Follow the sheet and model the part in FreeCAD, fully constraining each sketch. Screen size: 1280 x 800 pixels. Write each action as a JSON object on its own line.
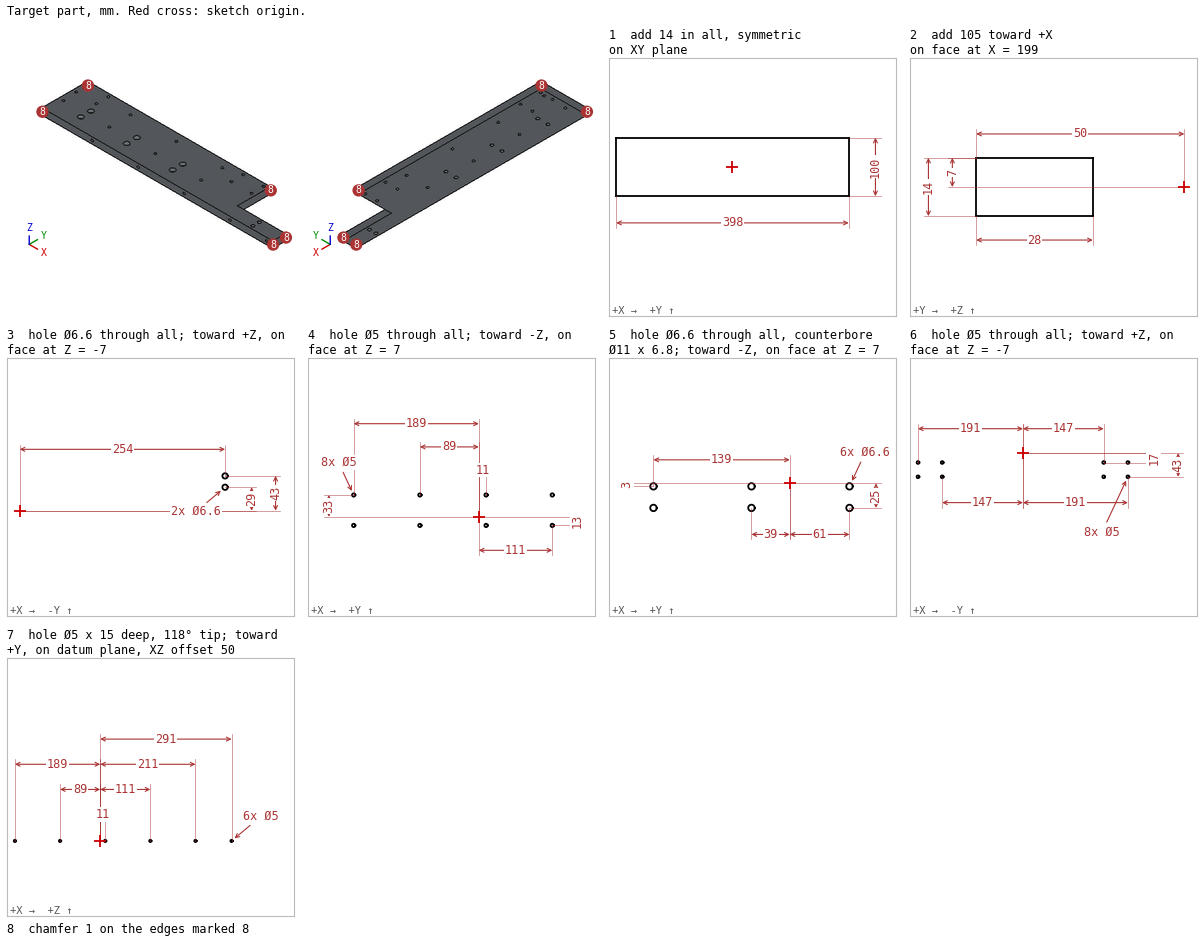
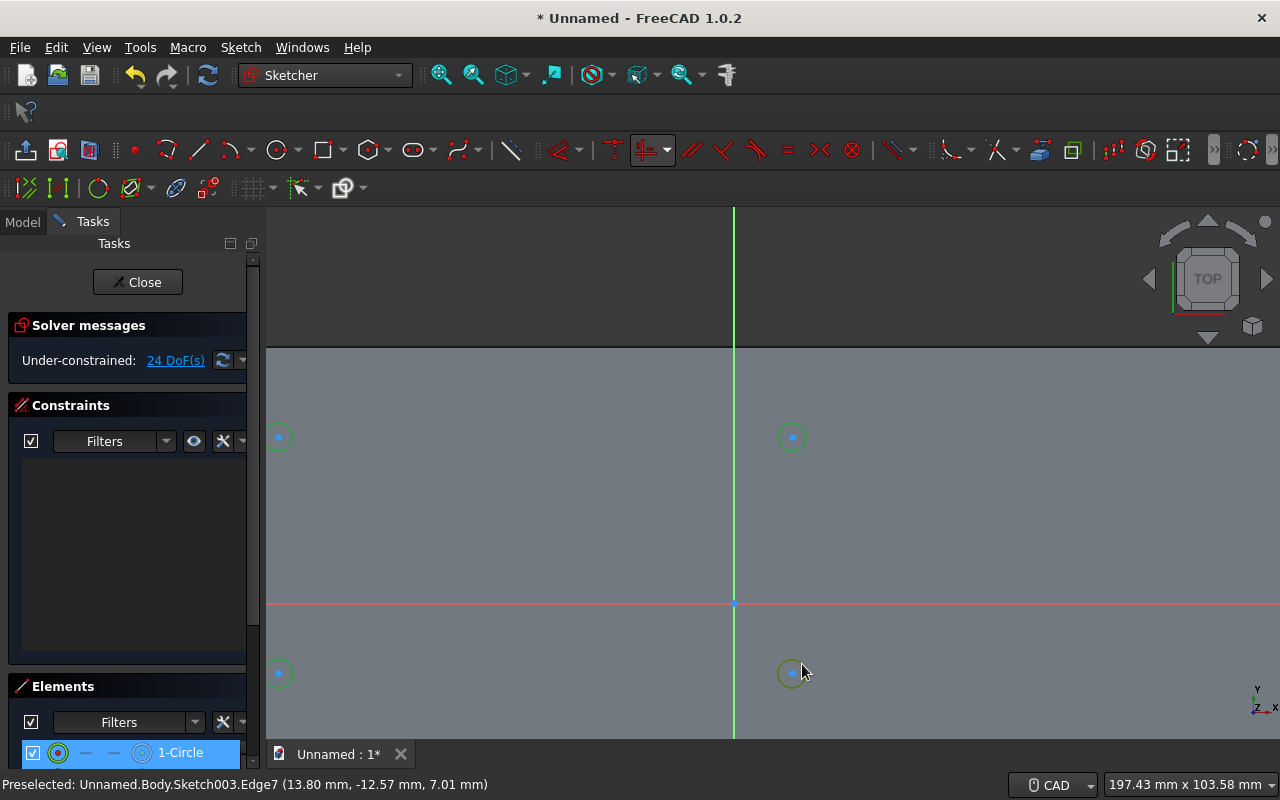
{"action": "scroll", "coordinate": [804, 427], "scroll_direction": "down", "scroll_amount": 5}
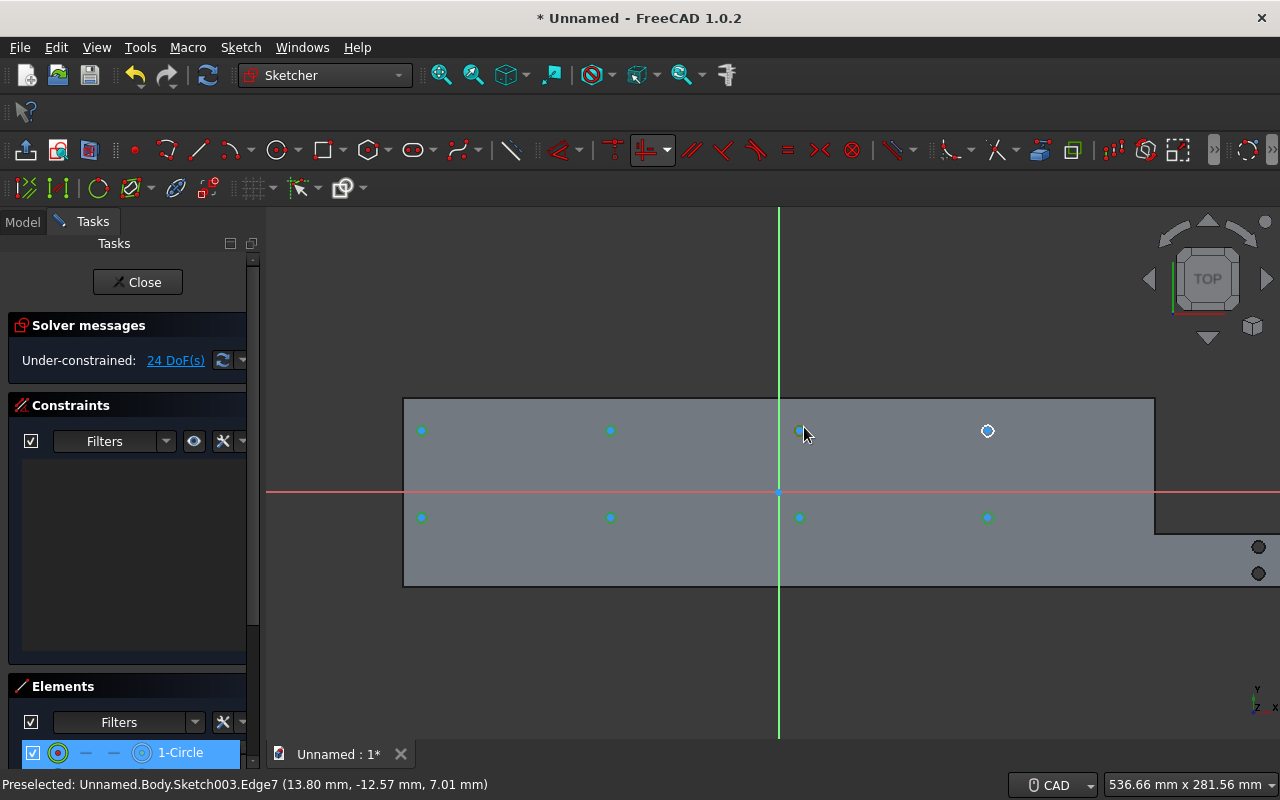
{"action": "scroll", "coordinate": [992, 427], "scroll_direction": "up", "scroll_amount": 5}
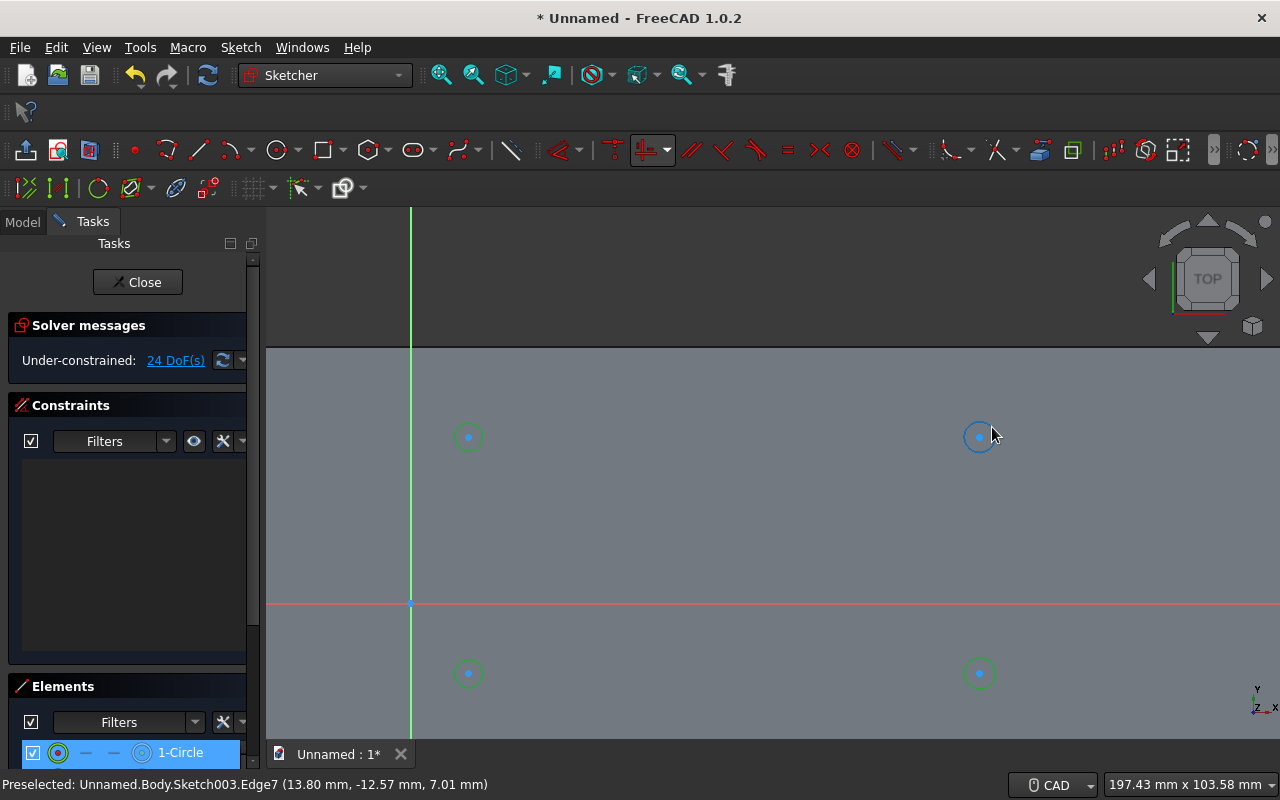
{"action": "left_click", "coordinate": [991, 426]}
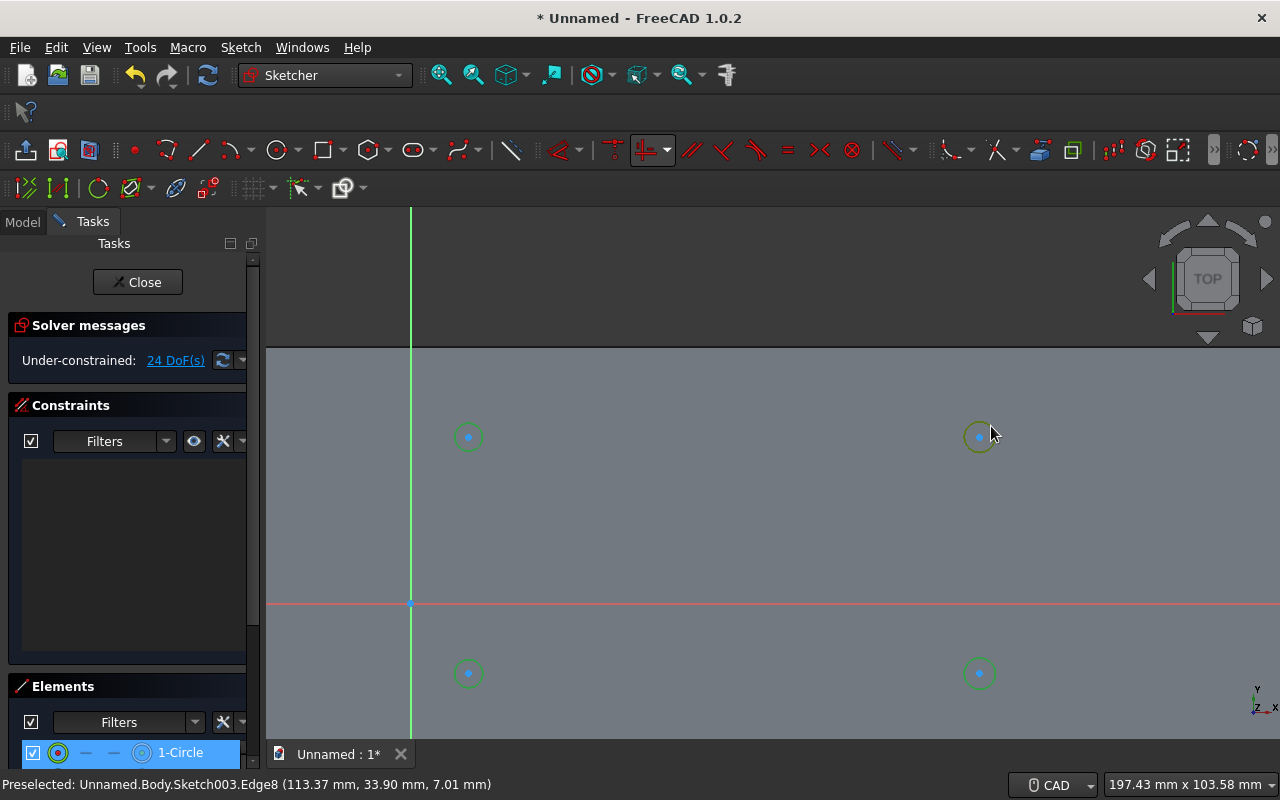
{"action": "key", "text": "e"}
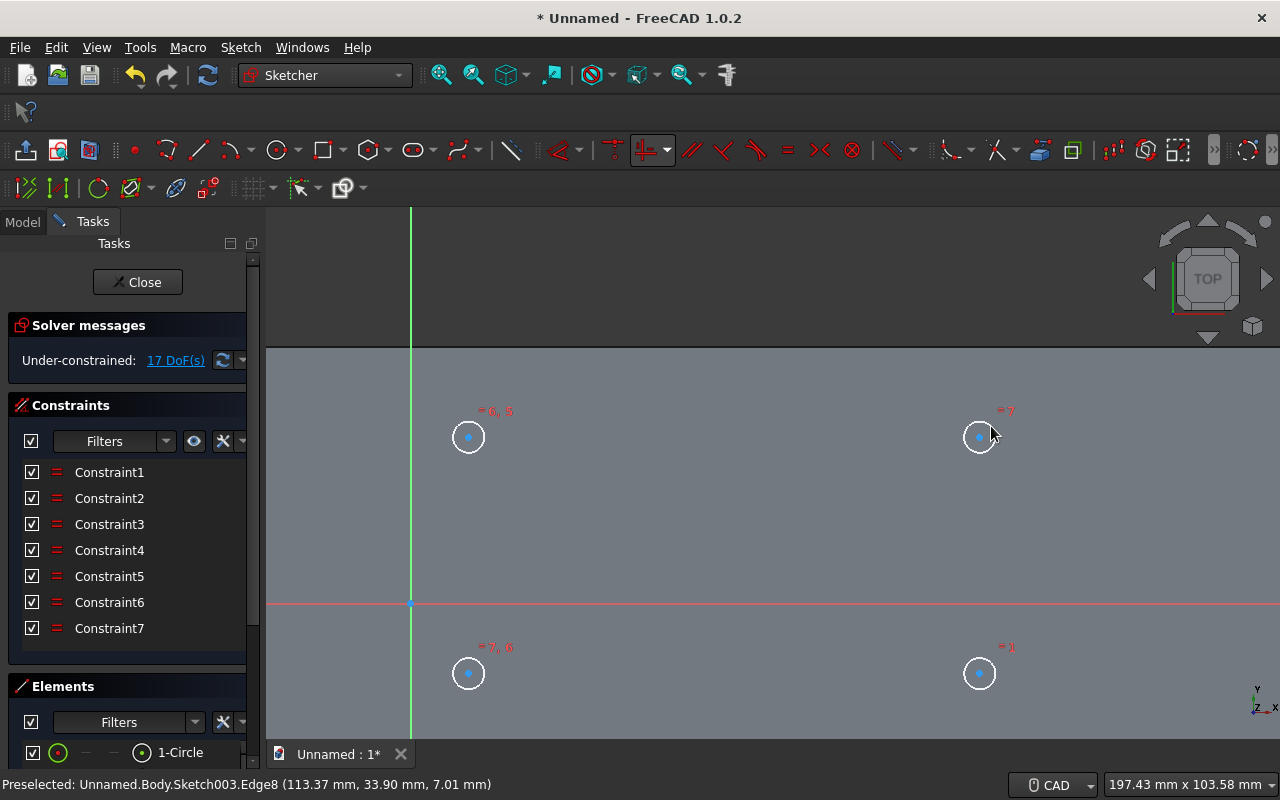
{"action": "scroll", "coordinate": [992, 427], "scroll_direction": "down", "scroll_amount": 5}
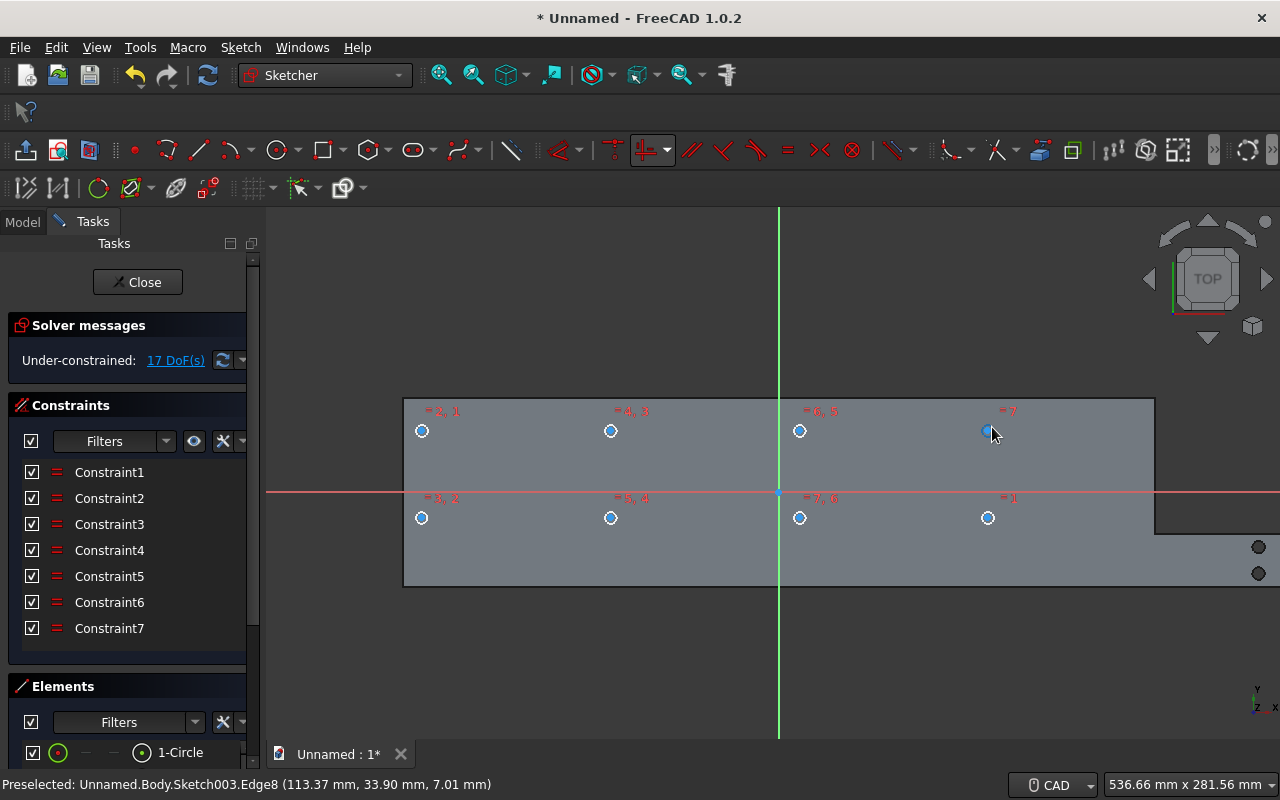
{"action": "left_click", "coordinate": [422, 431]}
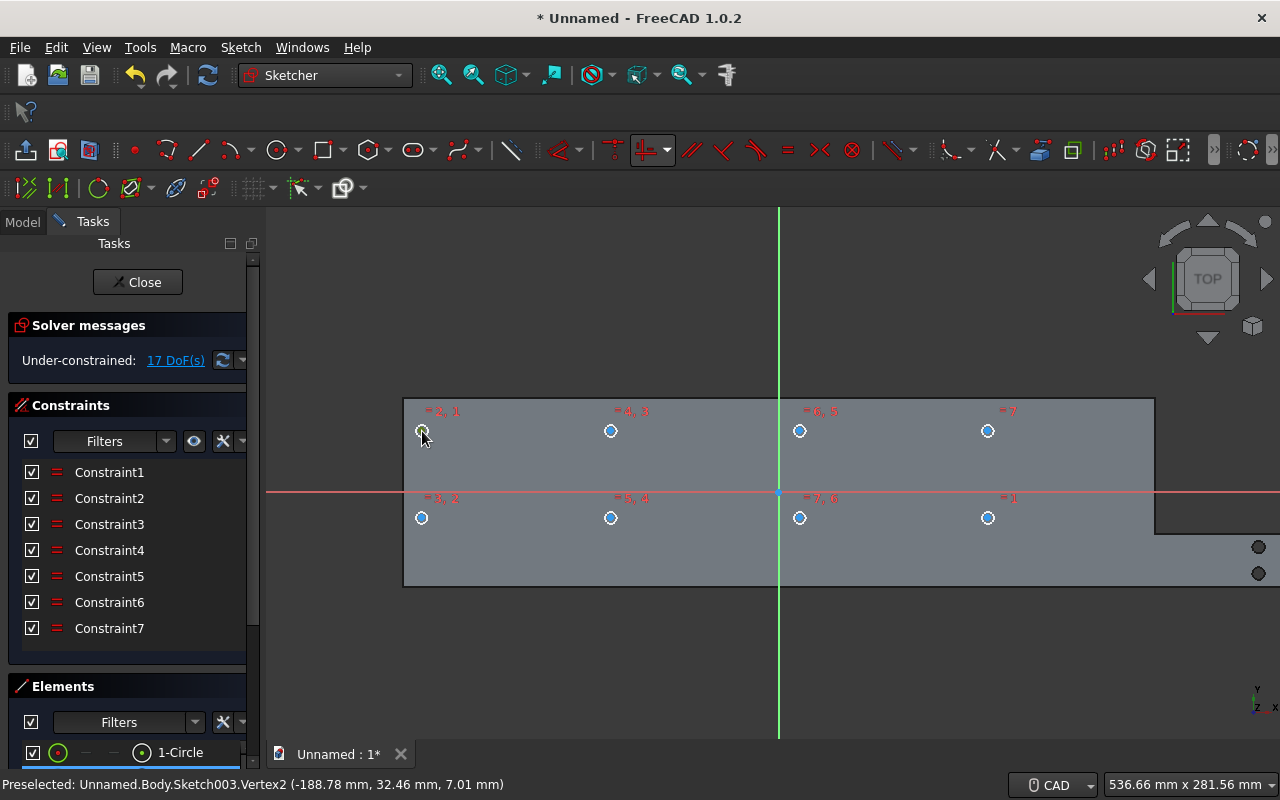
{"action": "left_click", "coordinate": [422, 518]}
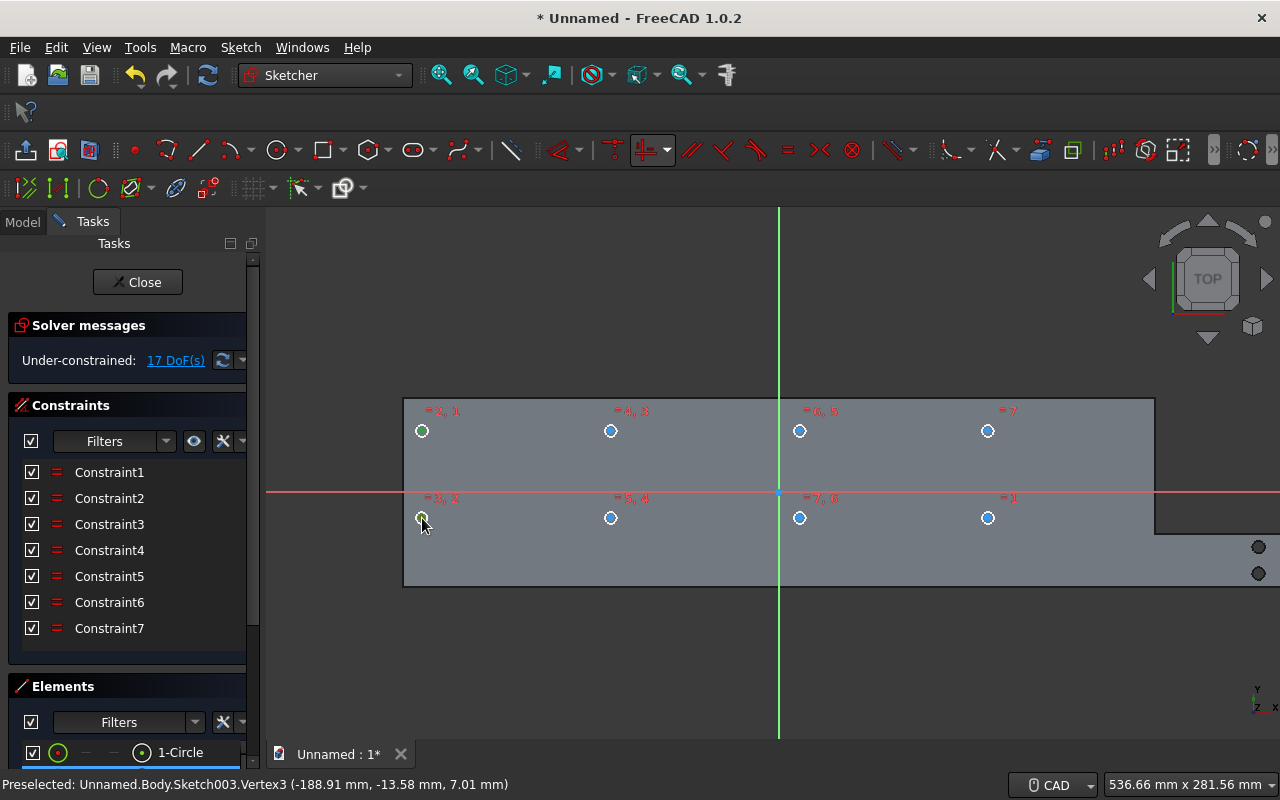
{"action": "key", "text": "v"}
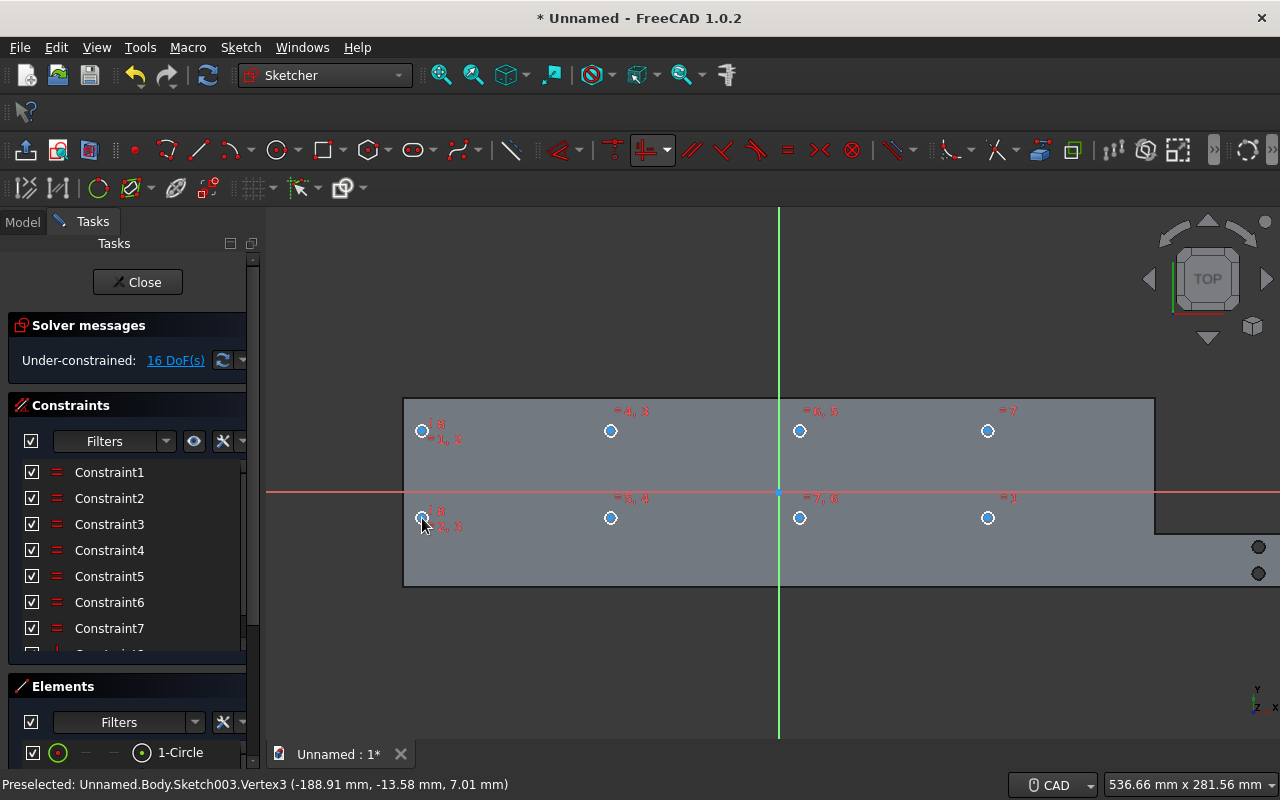
{"action": "left_click", "coordinate": [988, 518]}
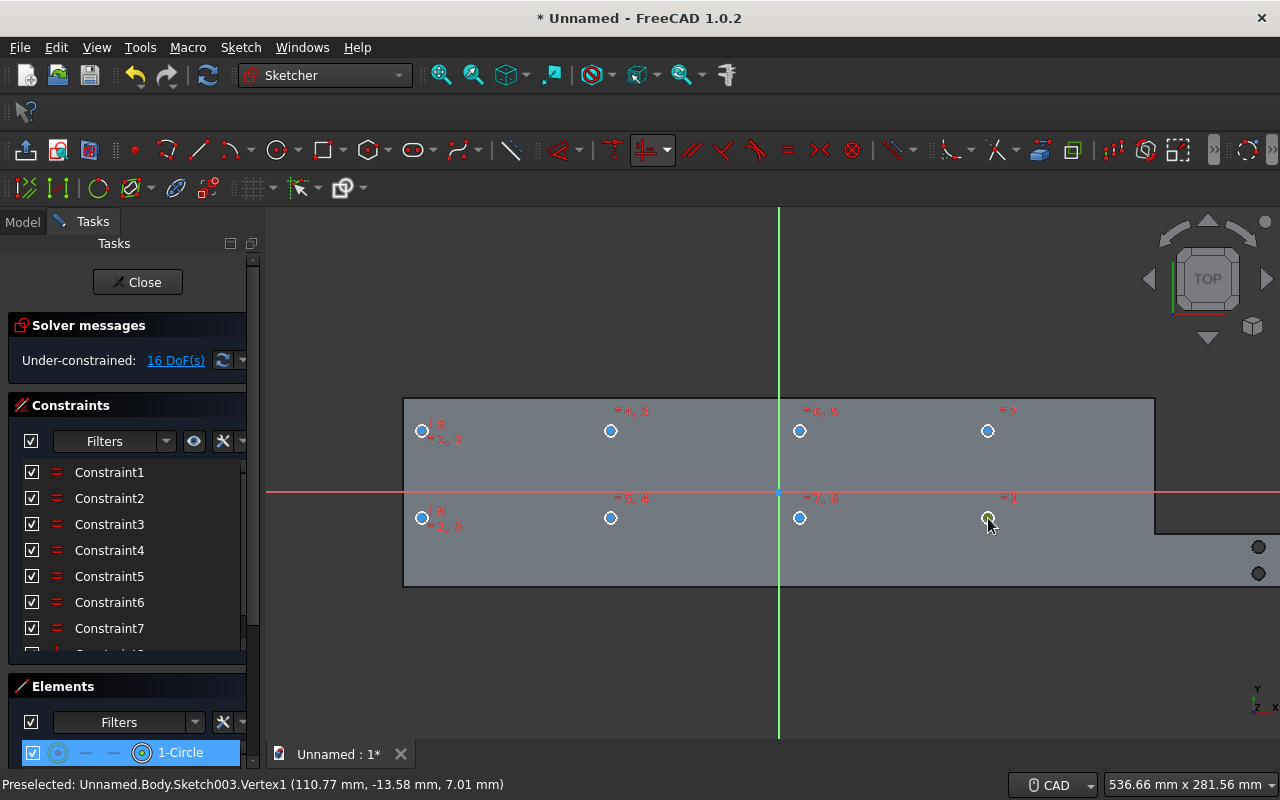
{"action": "left_click", "coordinate": [422, 518]}